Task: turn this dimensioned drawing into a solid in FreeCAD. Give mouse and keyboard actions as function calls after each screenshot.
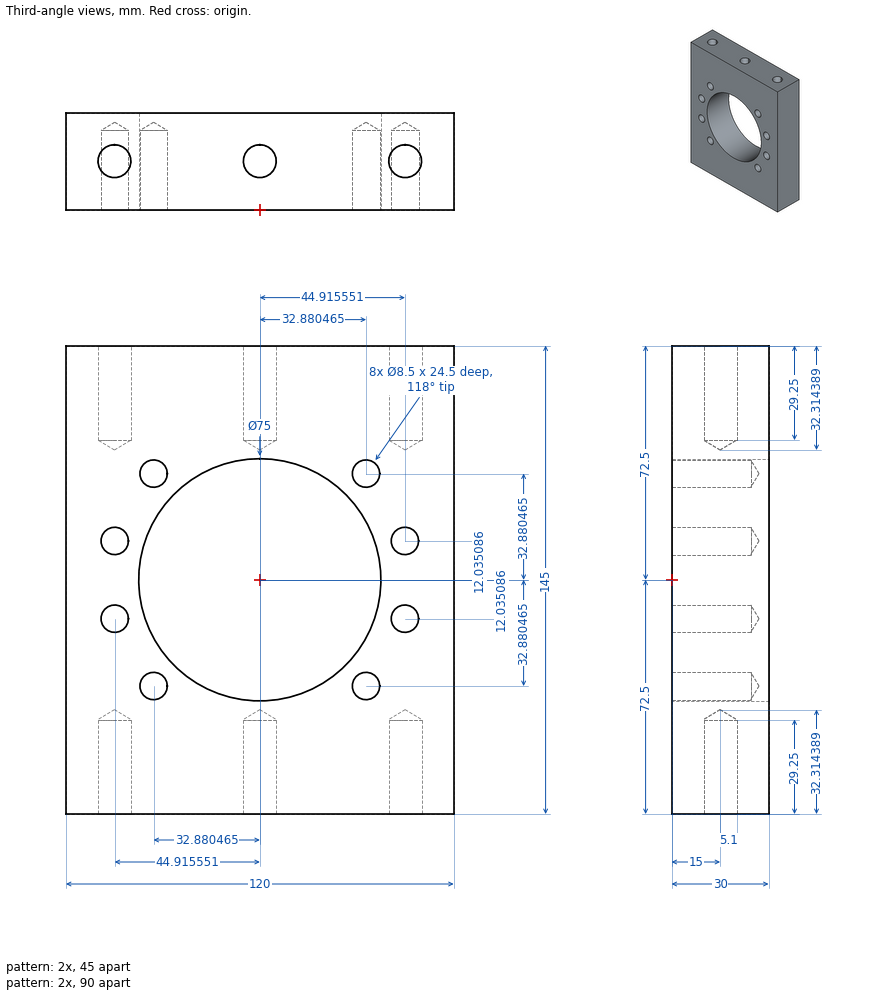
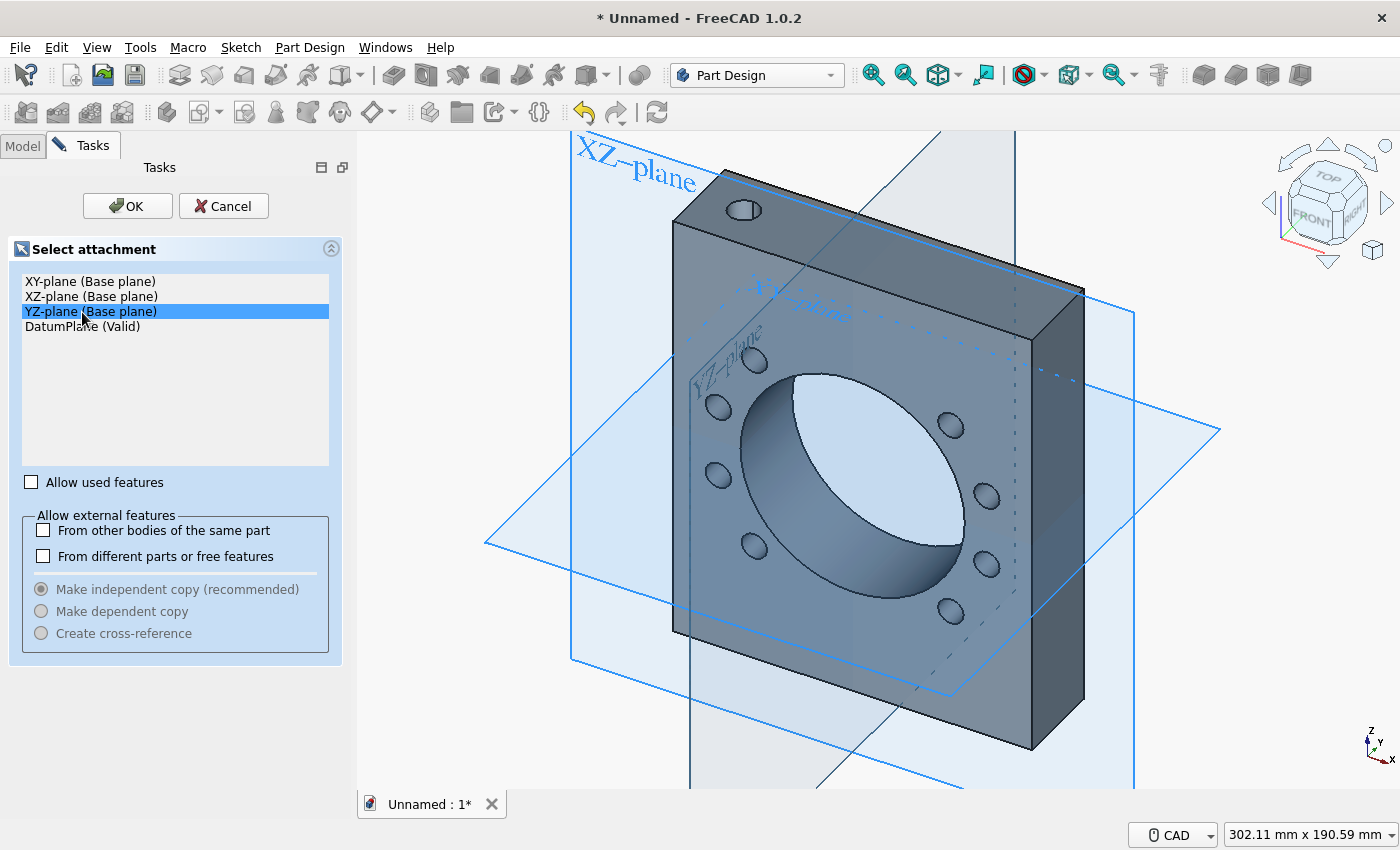
click(128, 206)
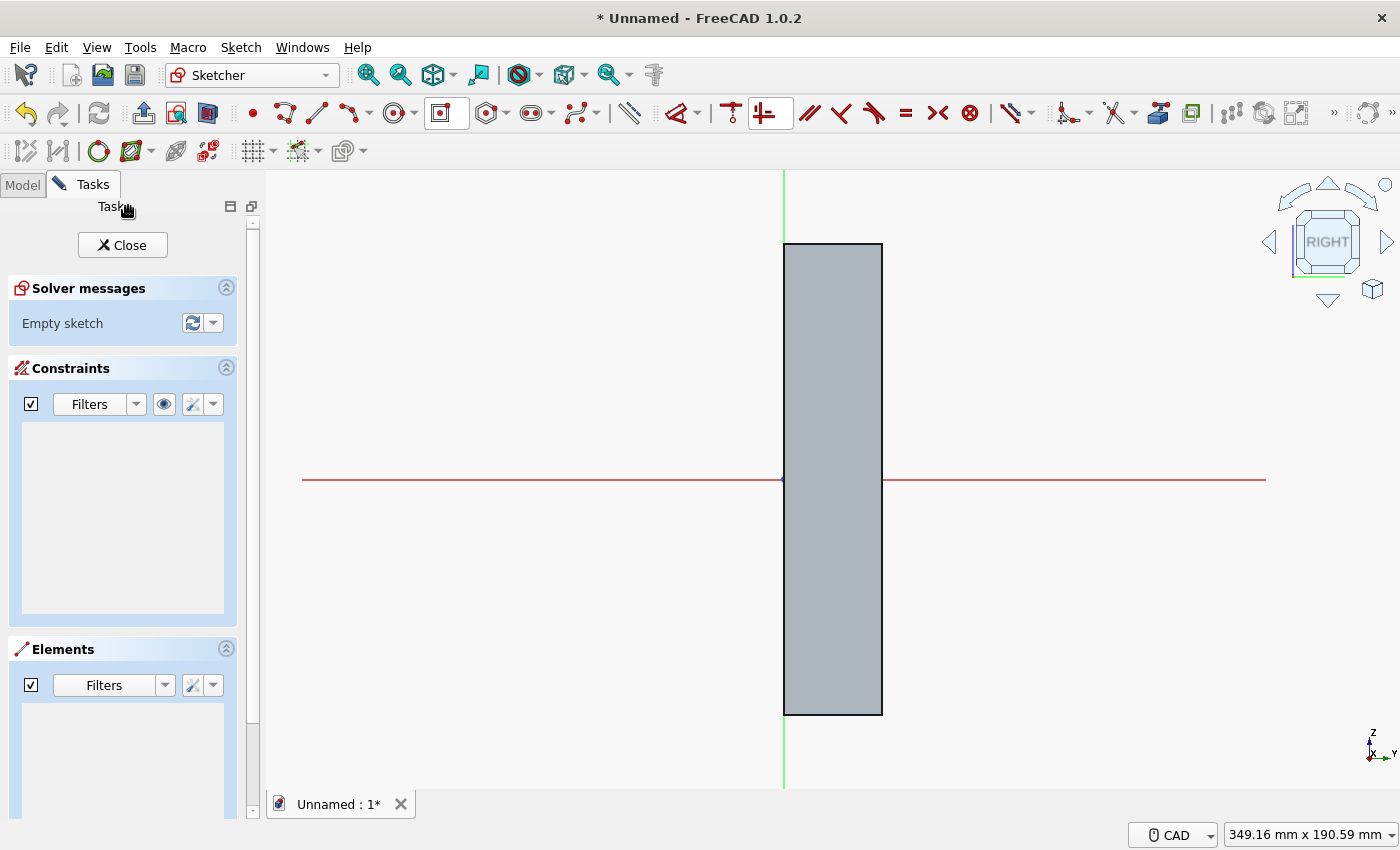
click(208, 114)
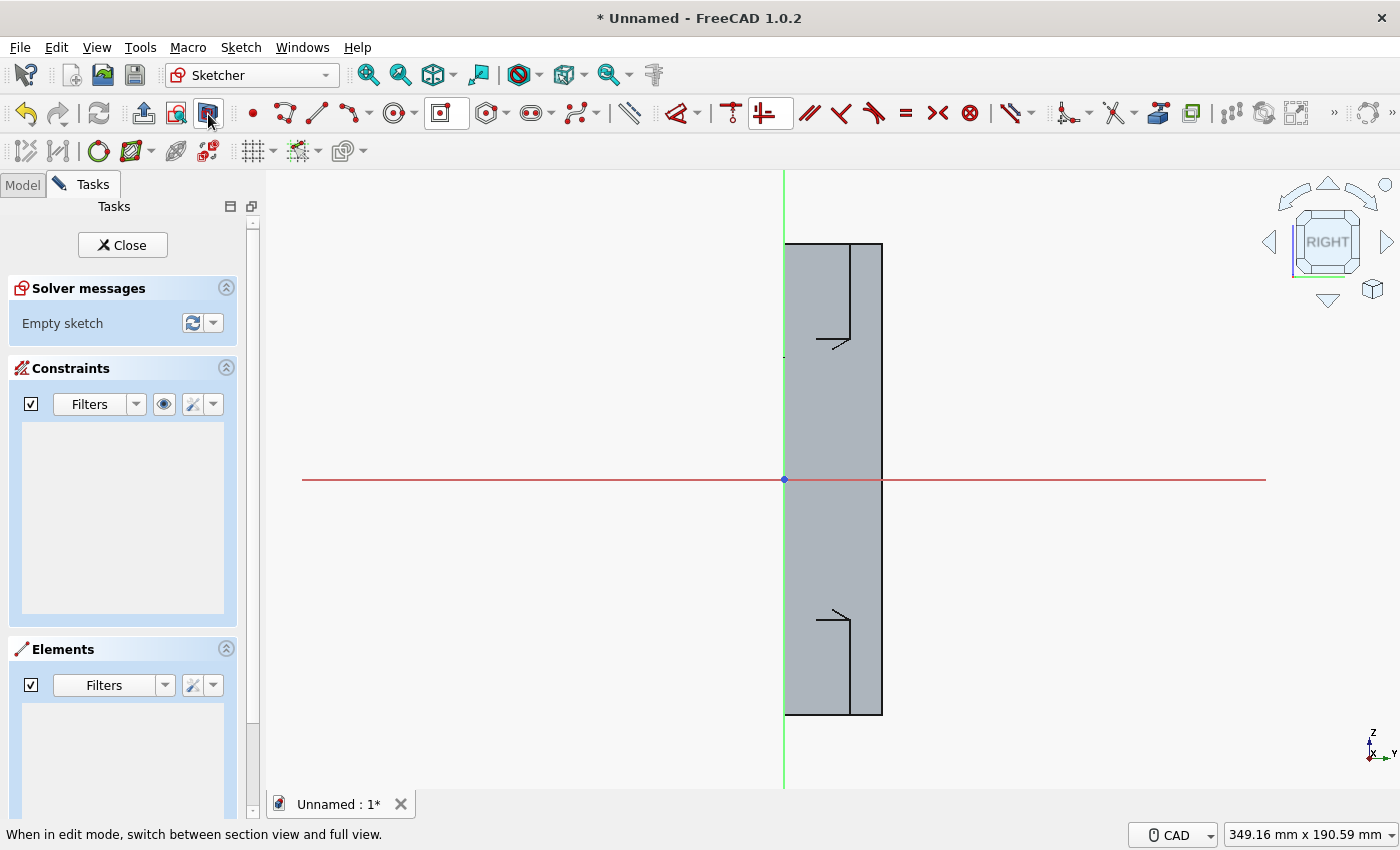
scroll(528, 761, down, 1)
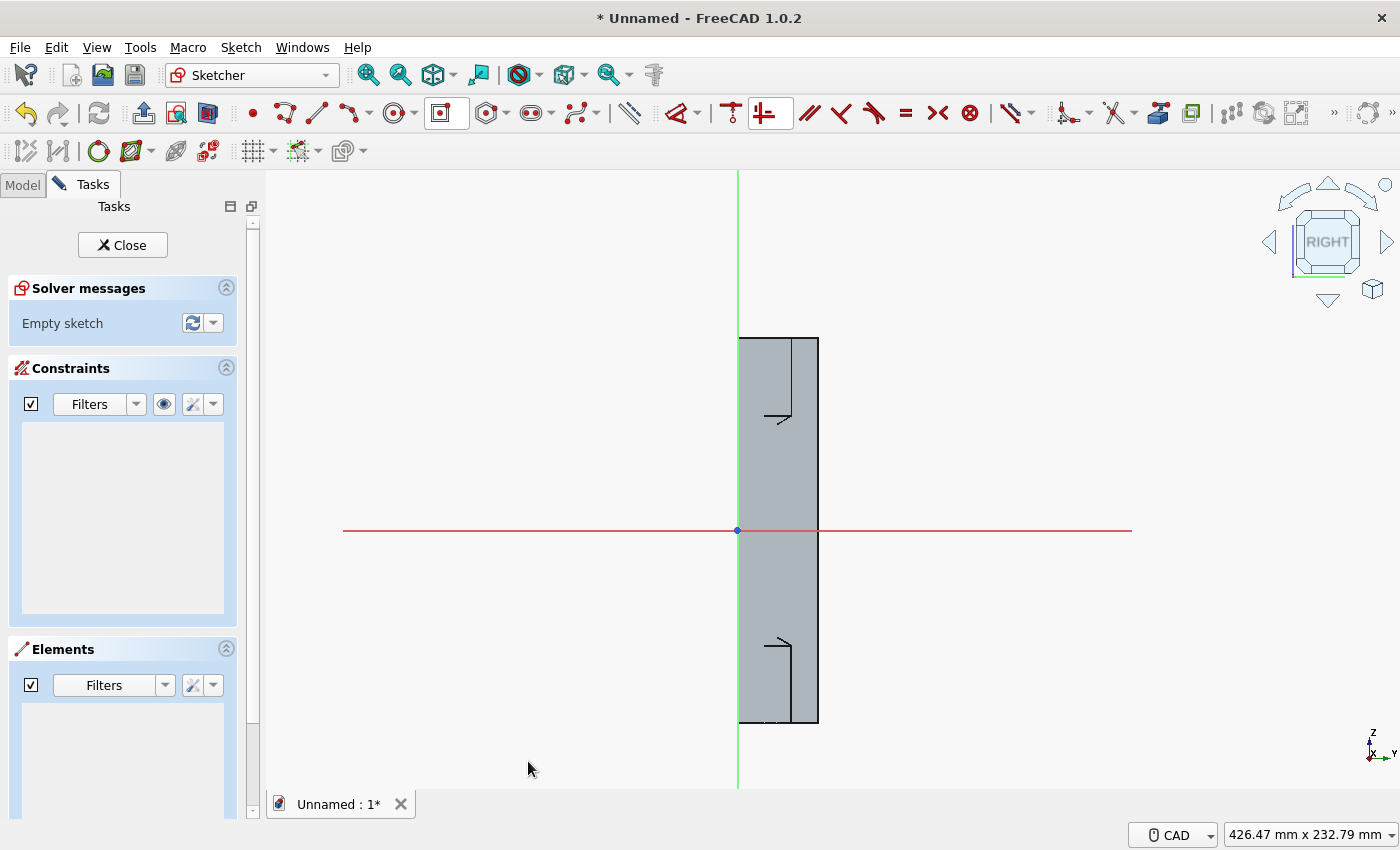
scroll(765, 341, up, 3)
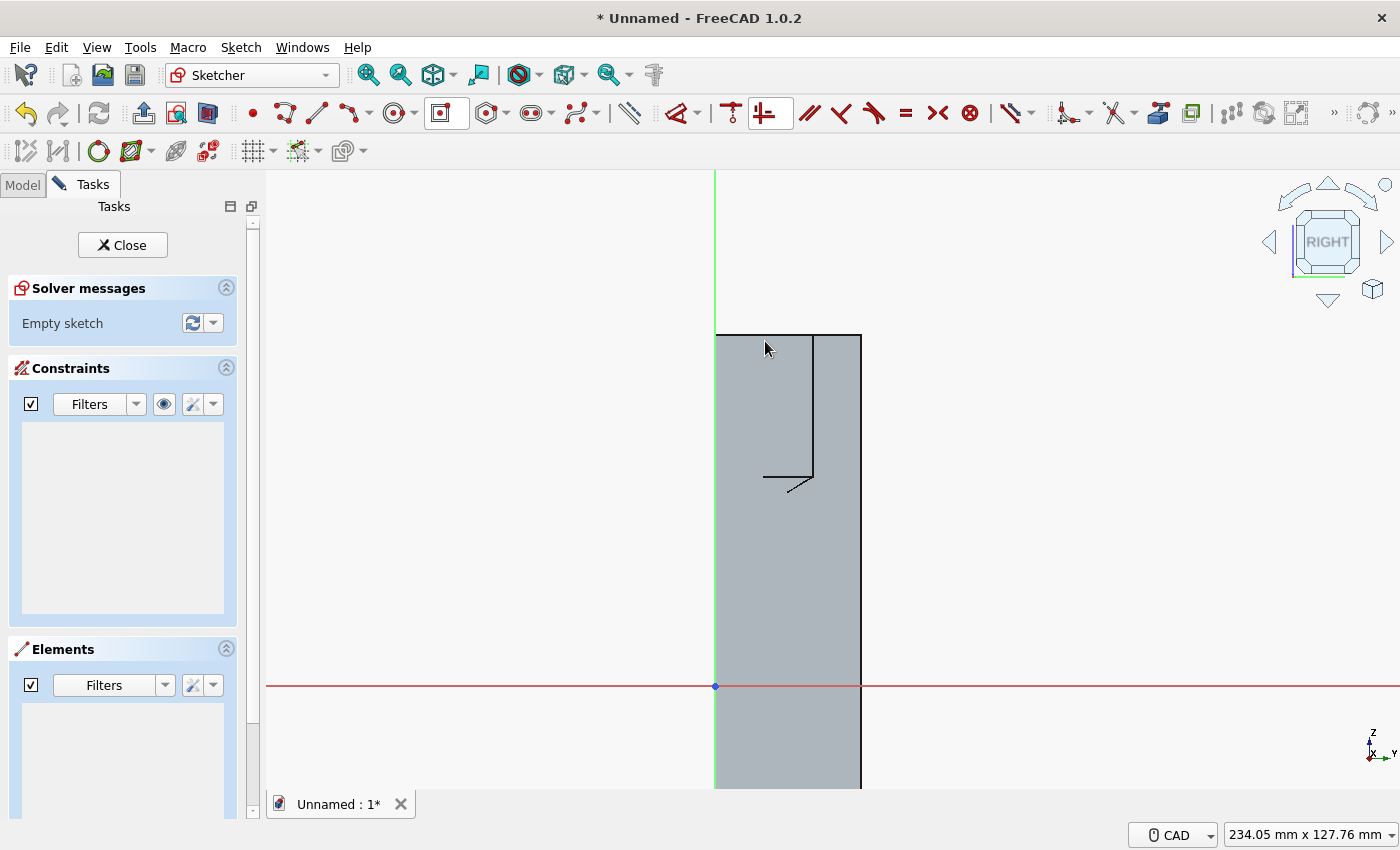
click(286, 114)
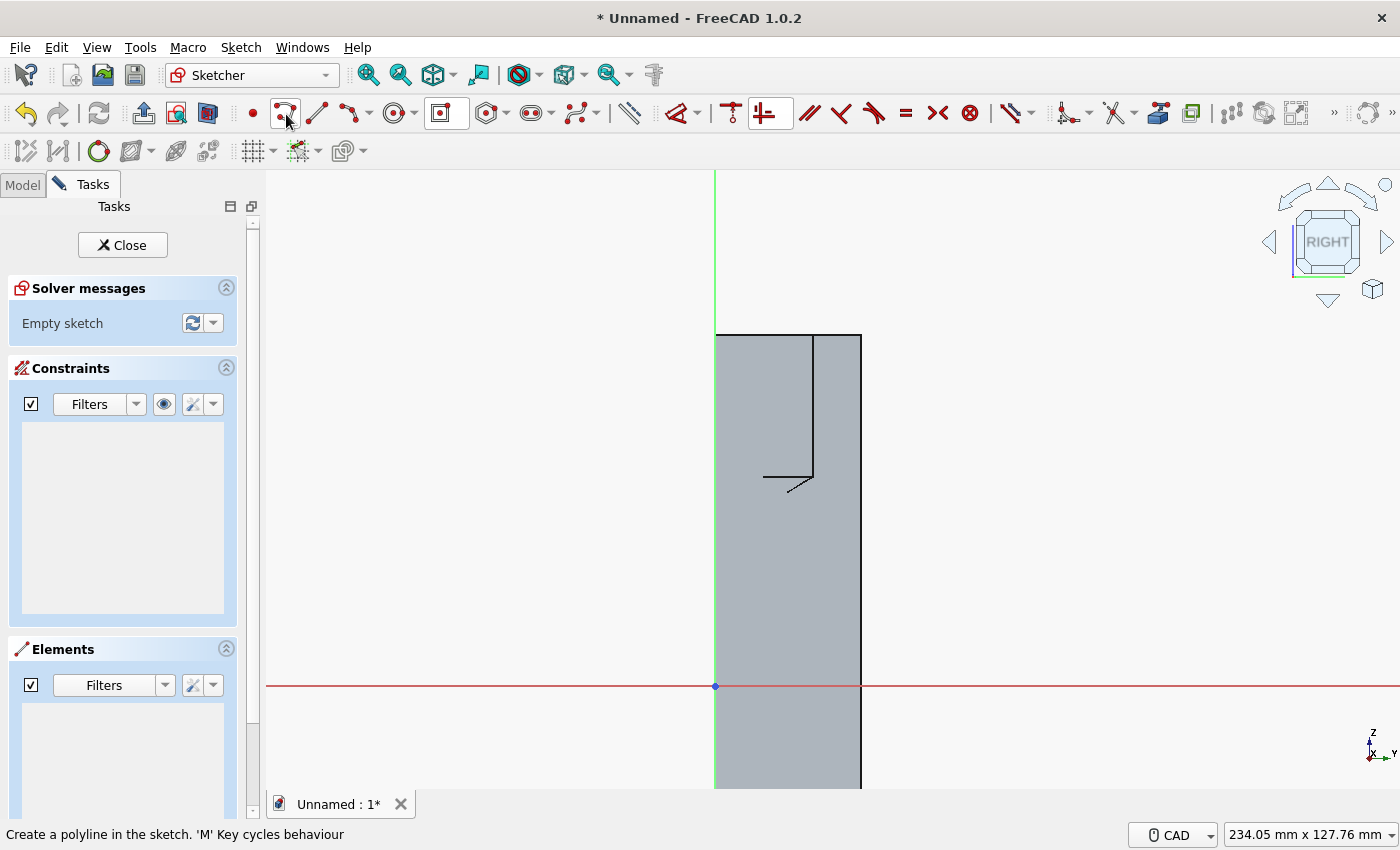
click(788, 492)
click(813, 477)
click(813, 335)
click(788, 335)
click(788, 493)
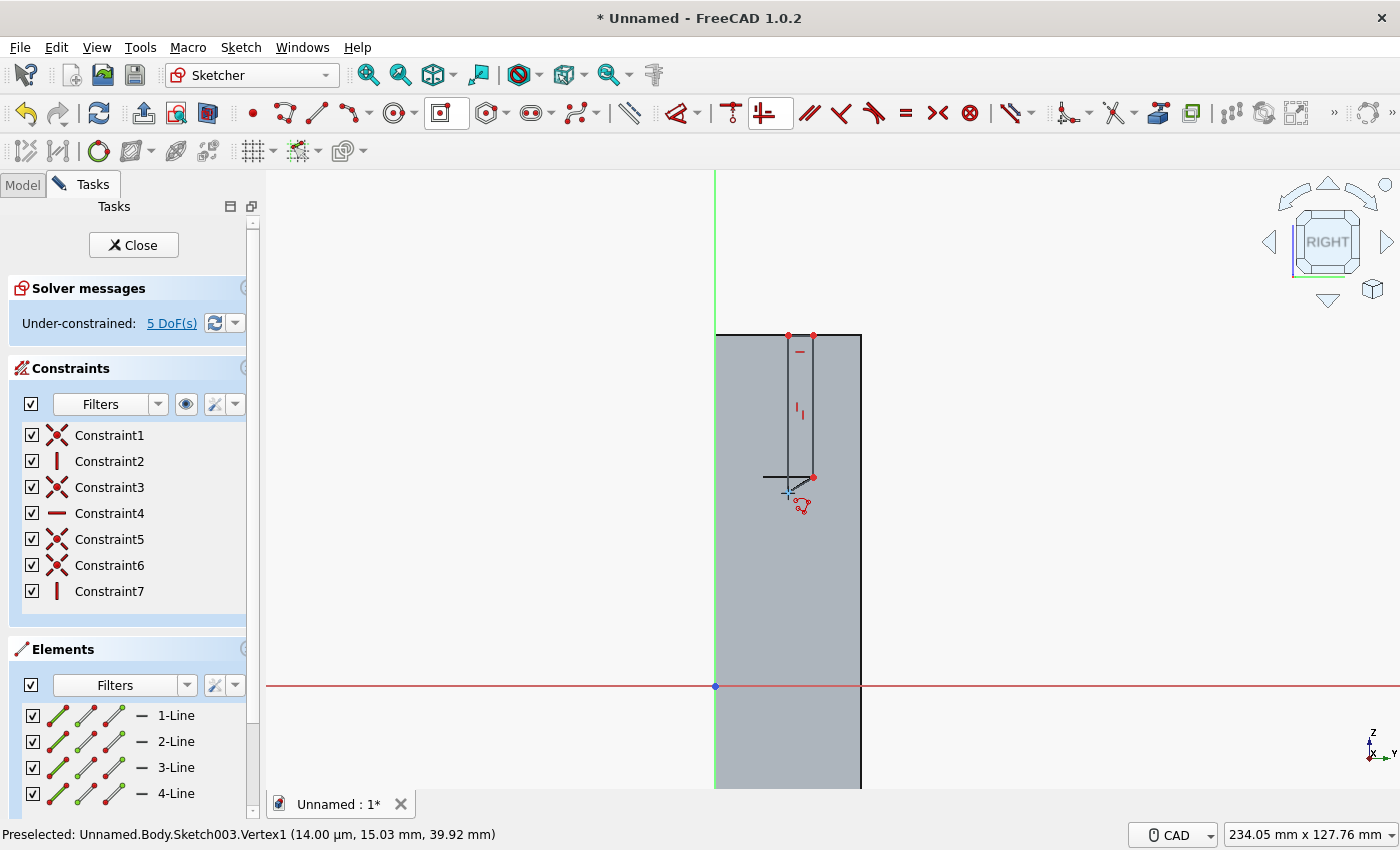
click(318, 114)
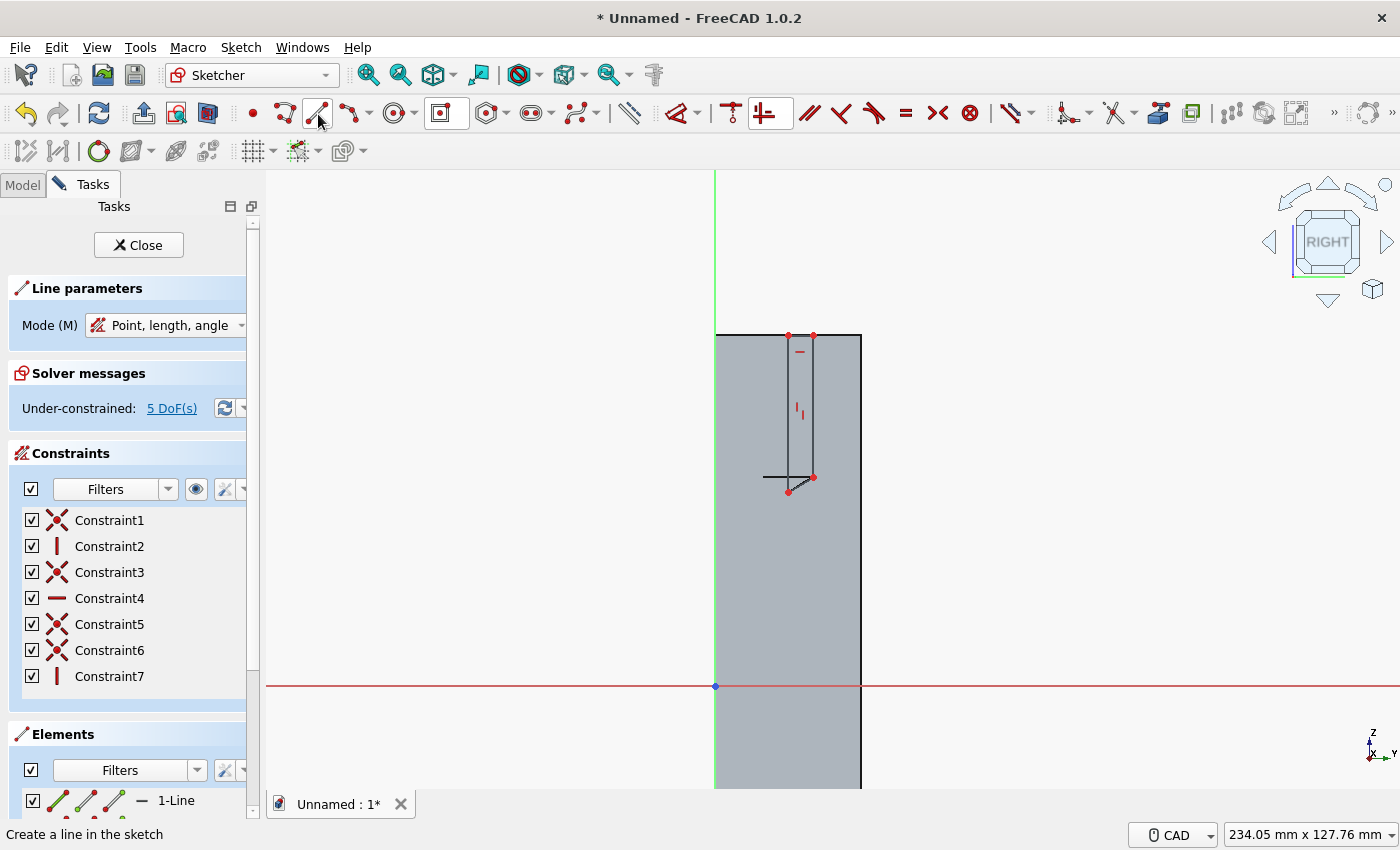
click(788, 320)
click(788, 273)
key(Escape)